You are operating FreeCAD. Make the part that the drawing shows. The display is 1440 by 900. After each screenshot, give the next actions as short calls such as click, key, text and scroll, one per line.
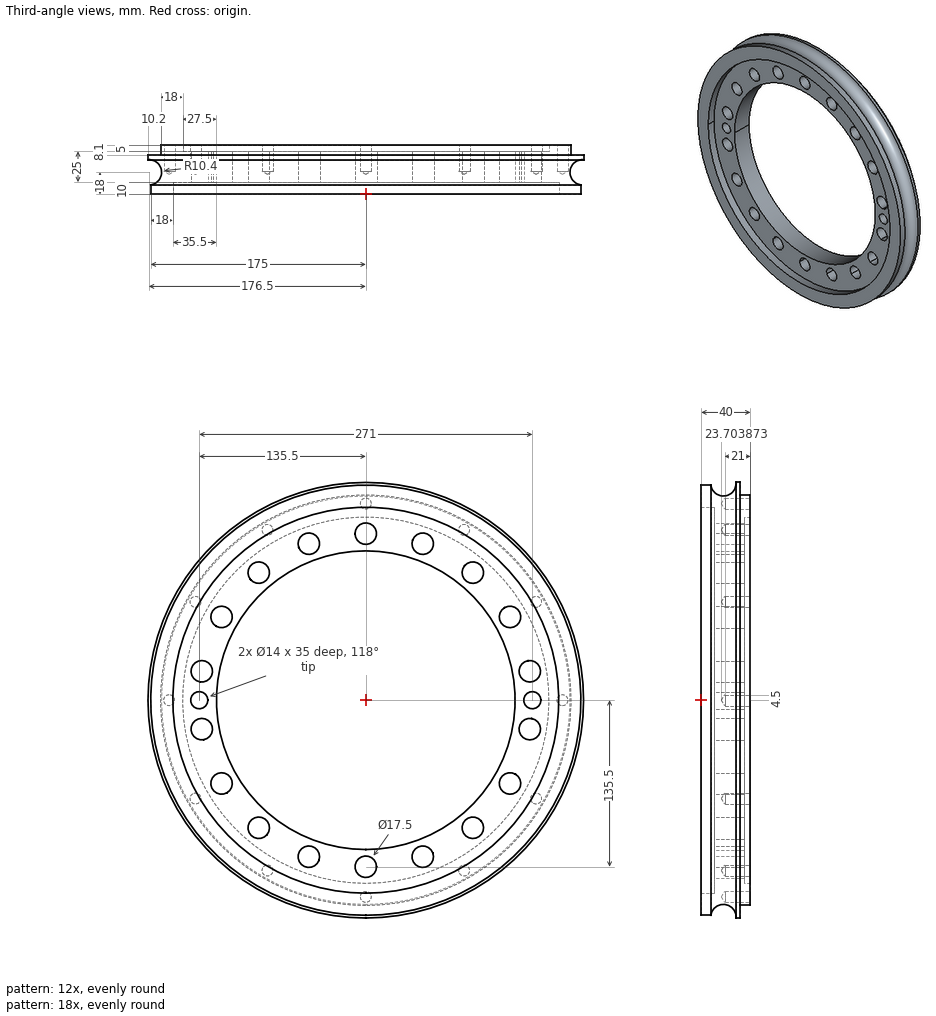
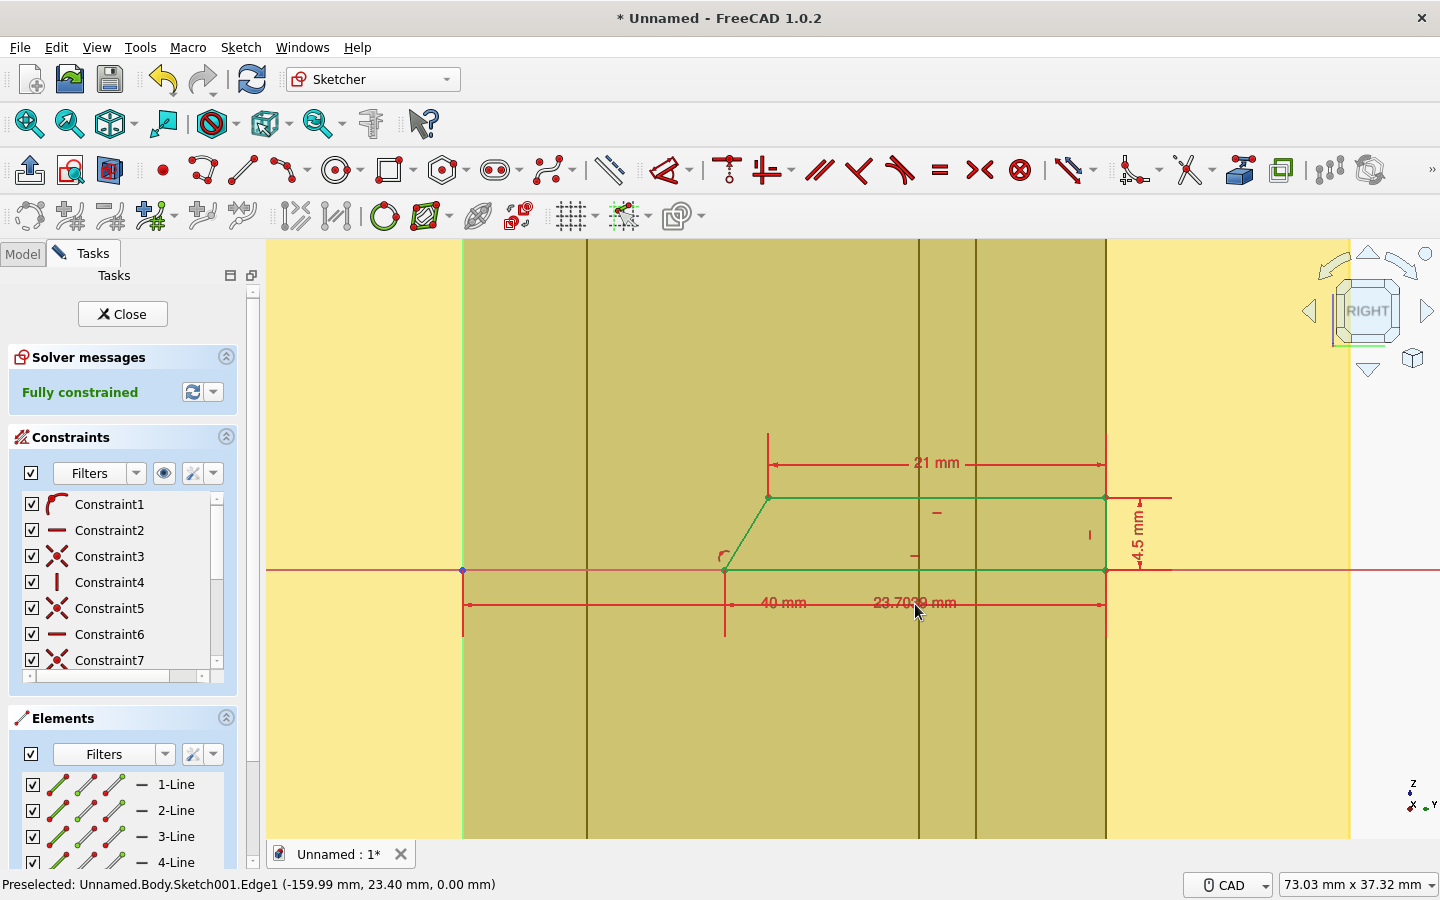
click(123, 314)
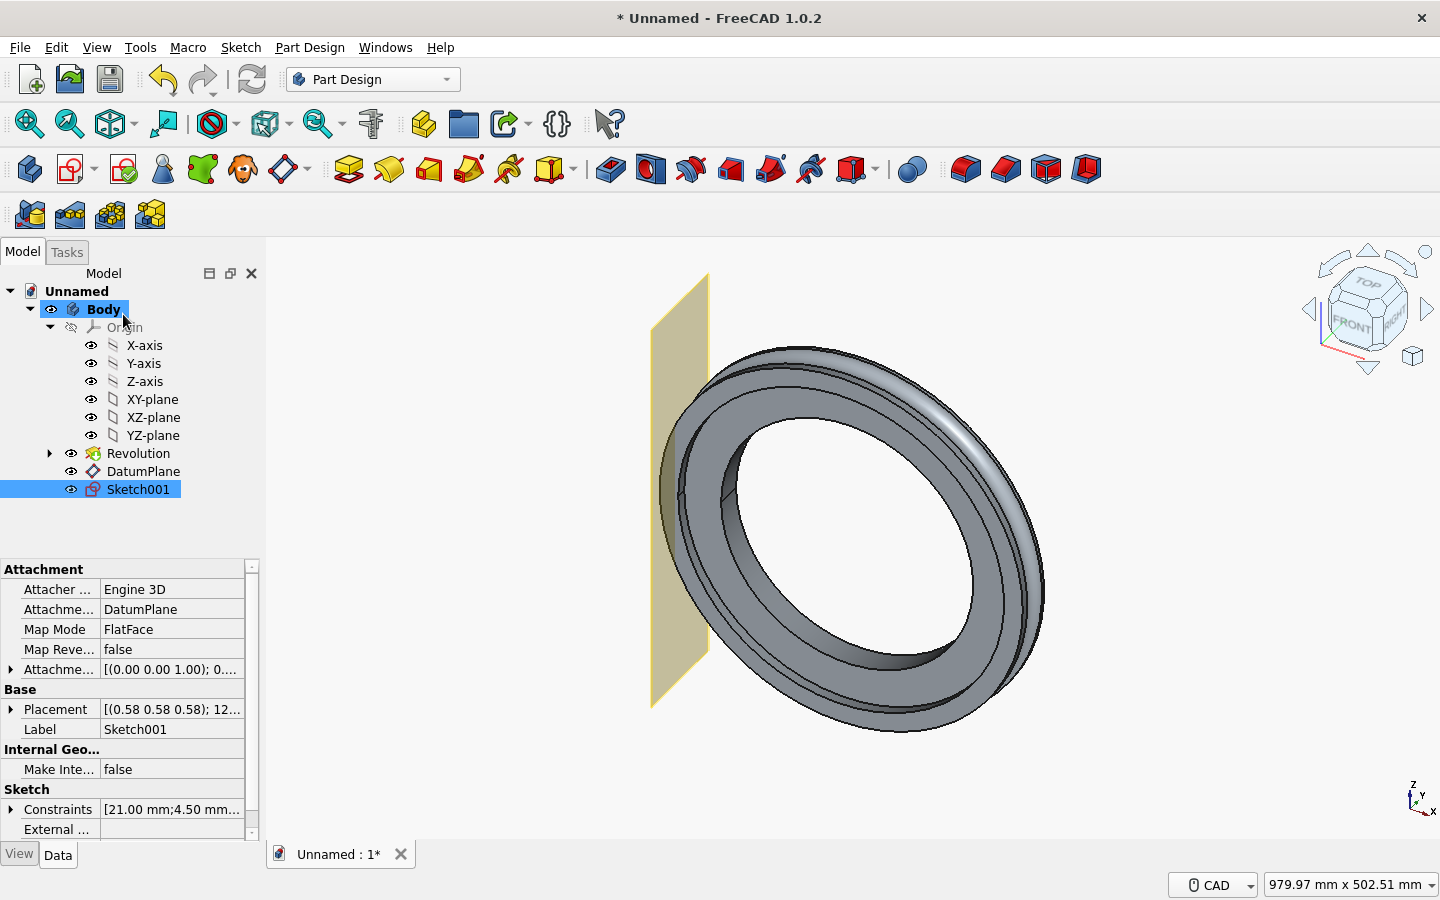
click(692, 170)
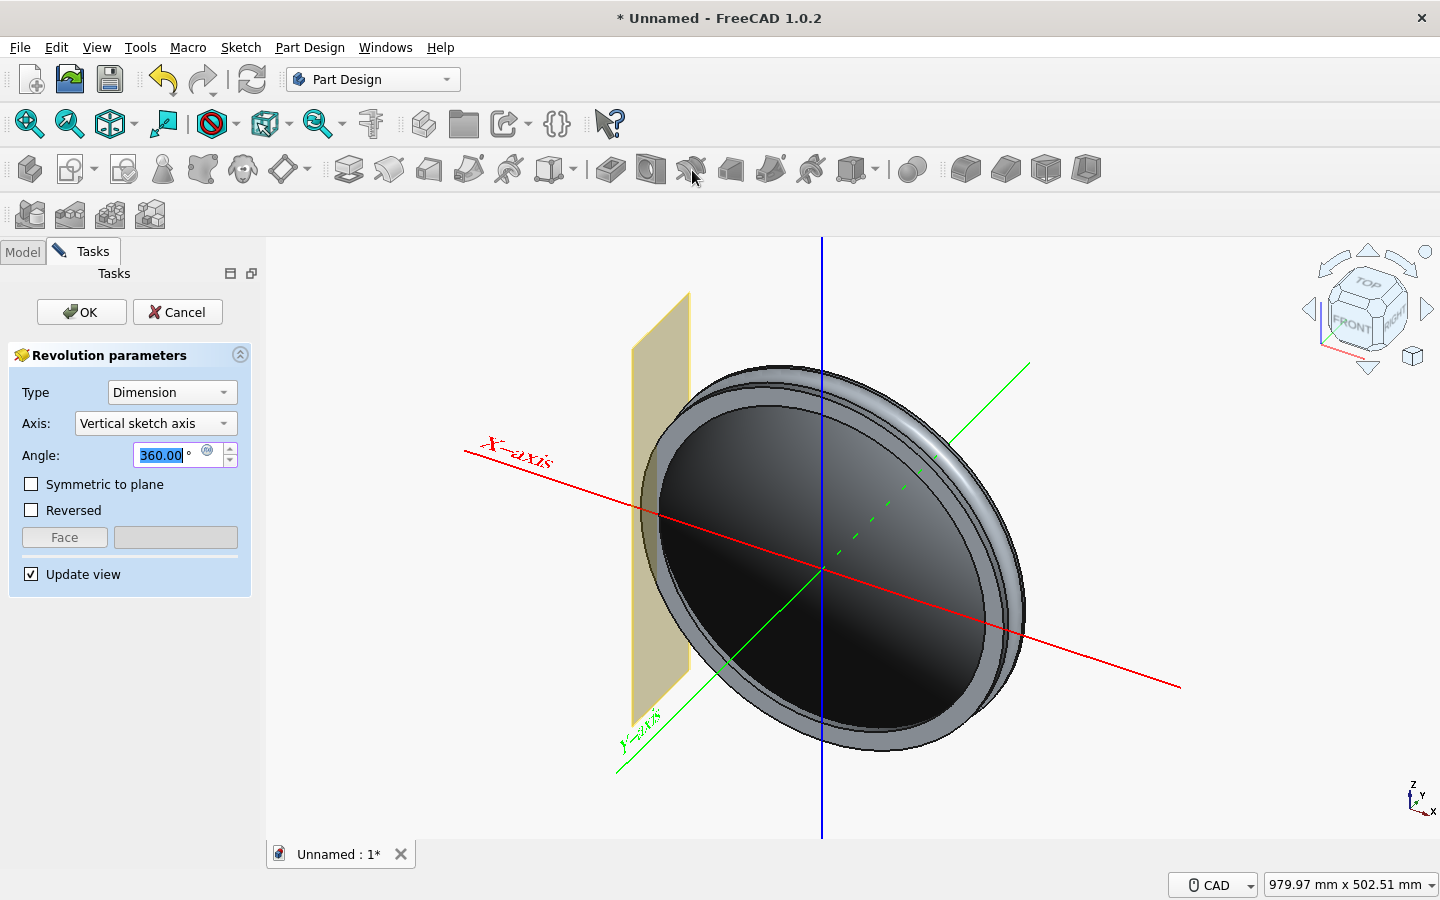
click(156, 424)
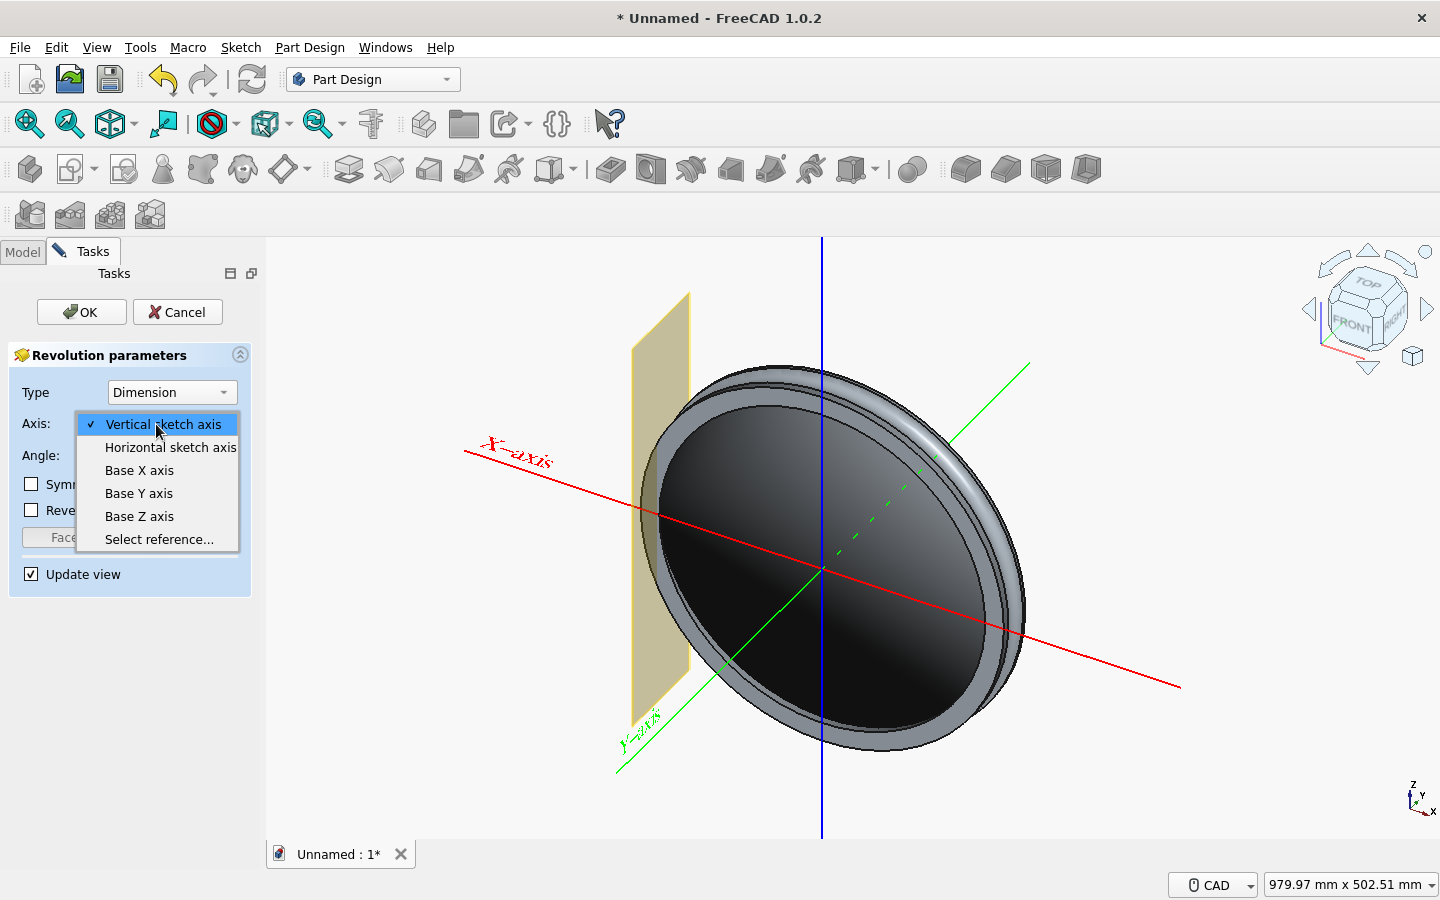
click(156, 448)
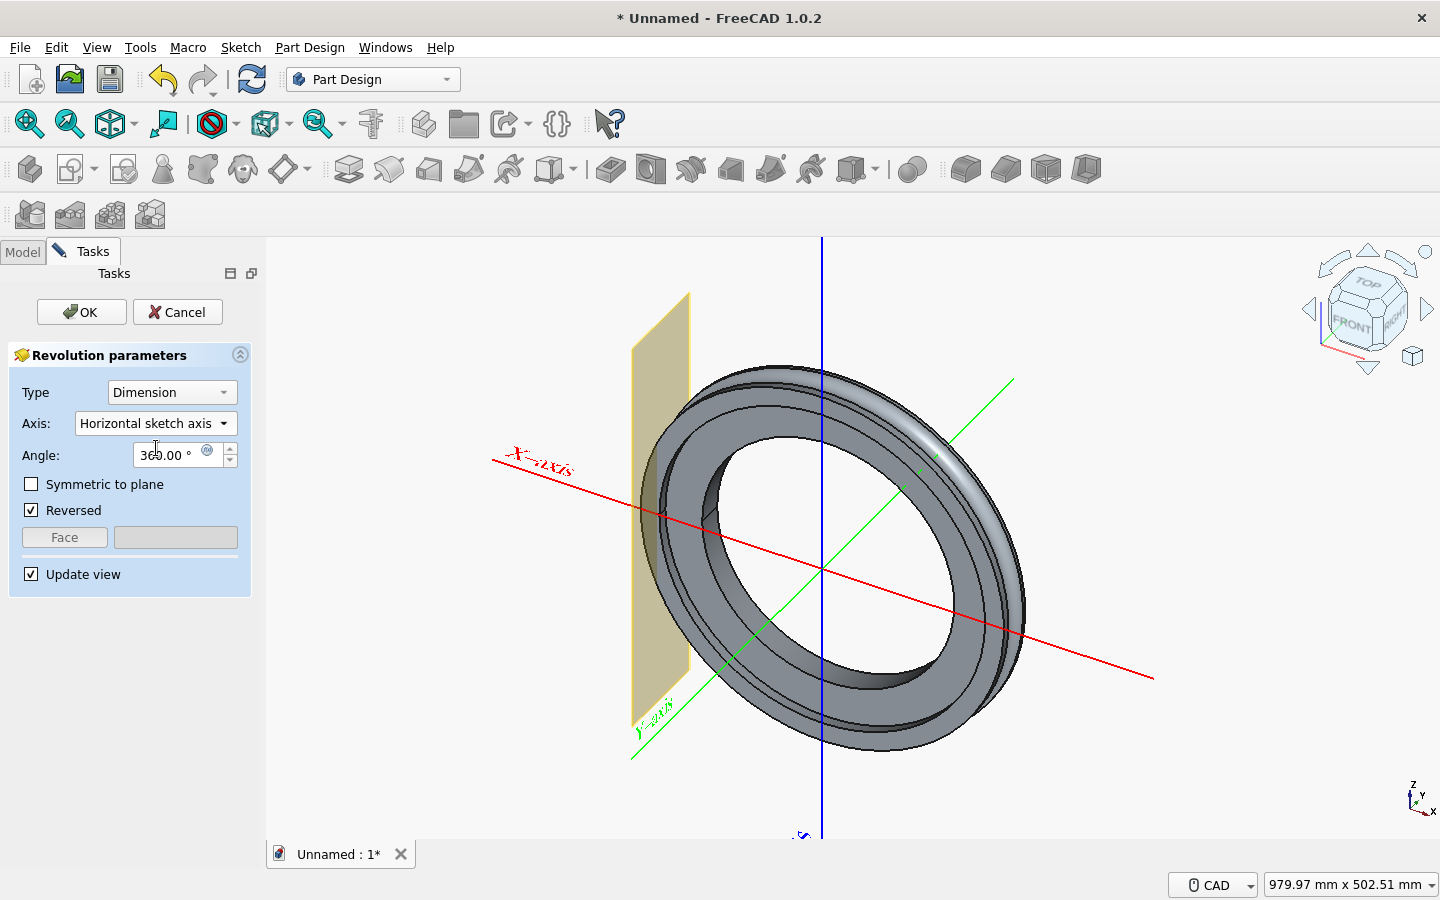
click(82, 312)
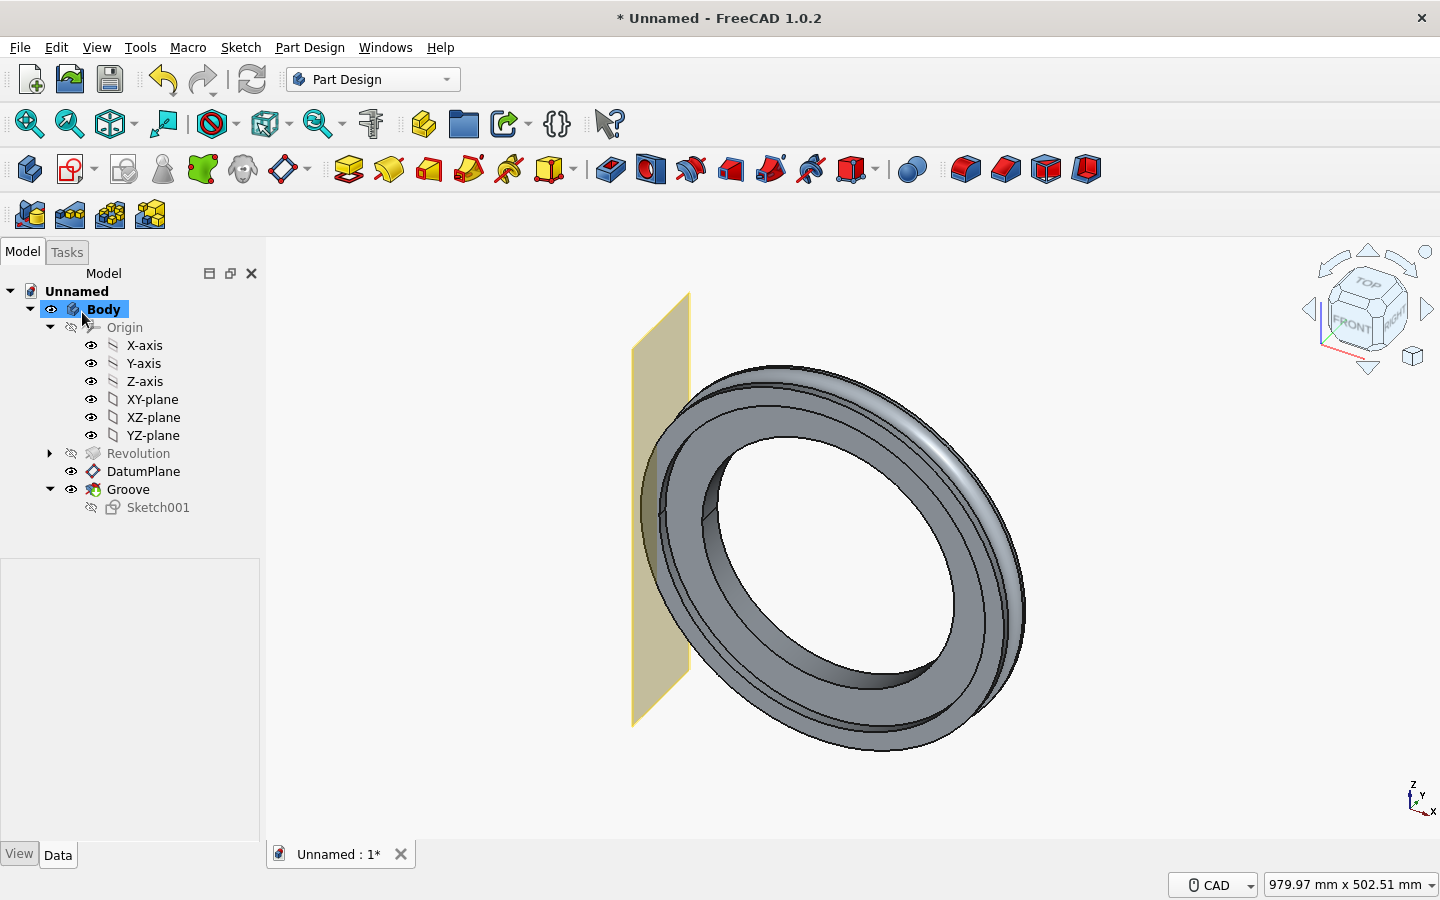
click(116, 471)
key(space)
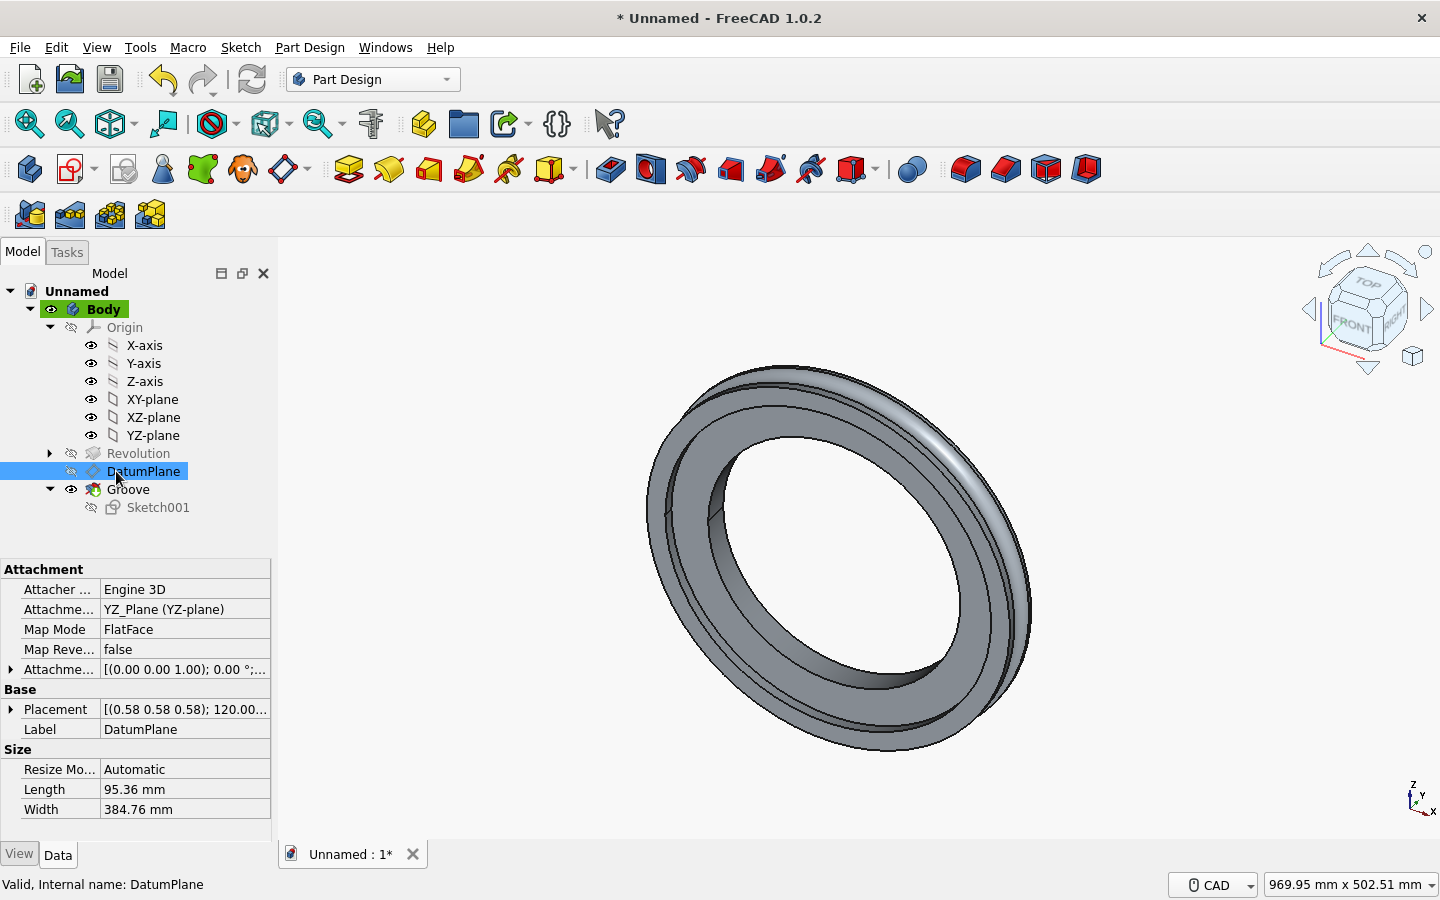
click(116, 489)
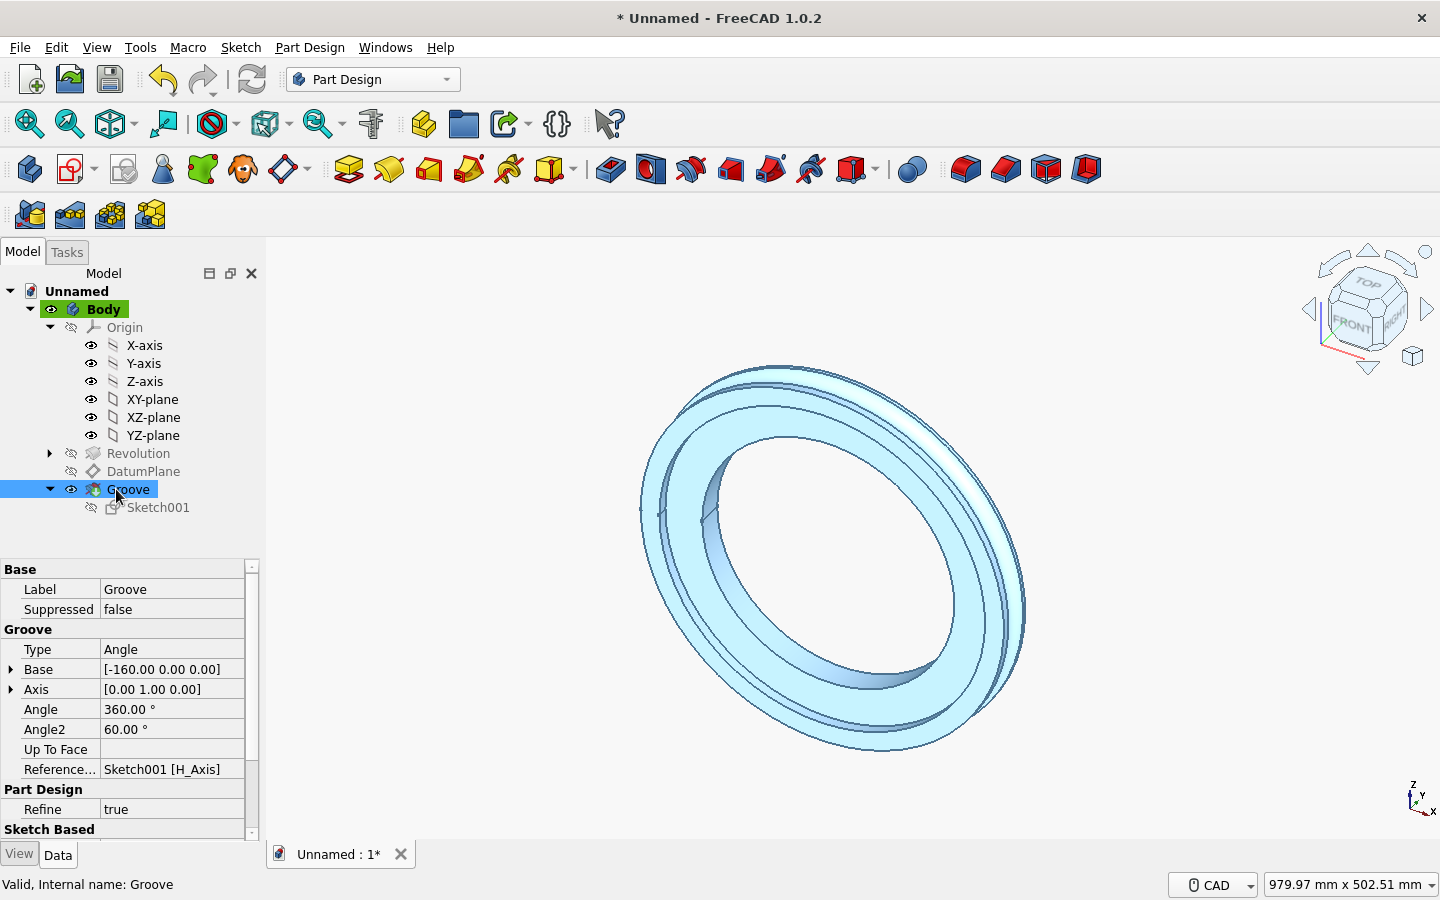
click(110, 214)